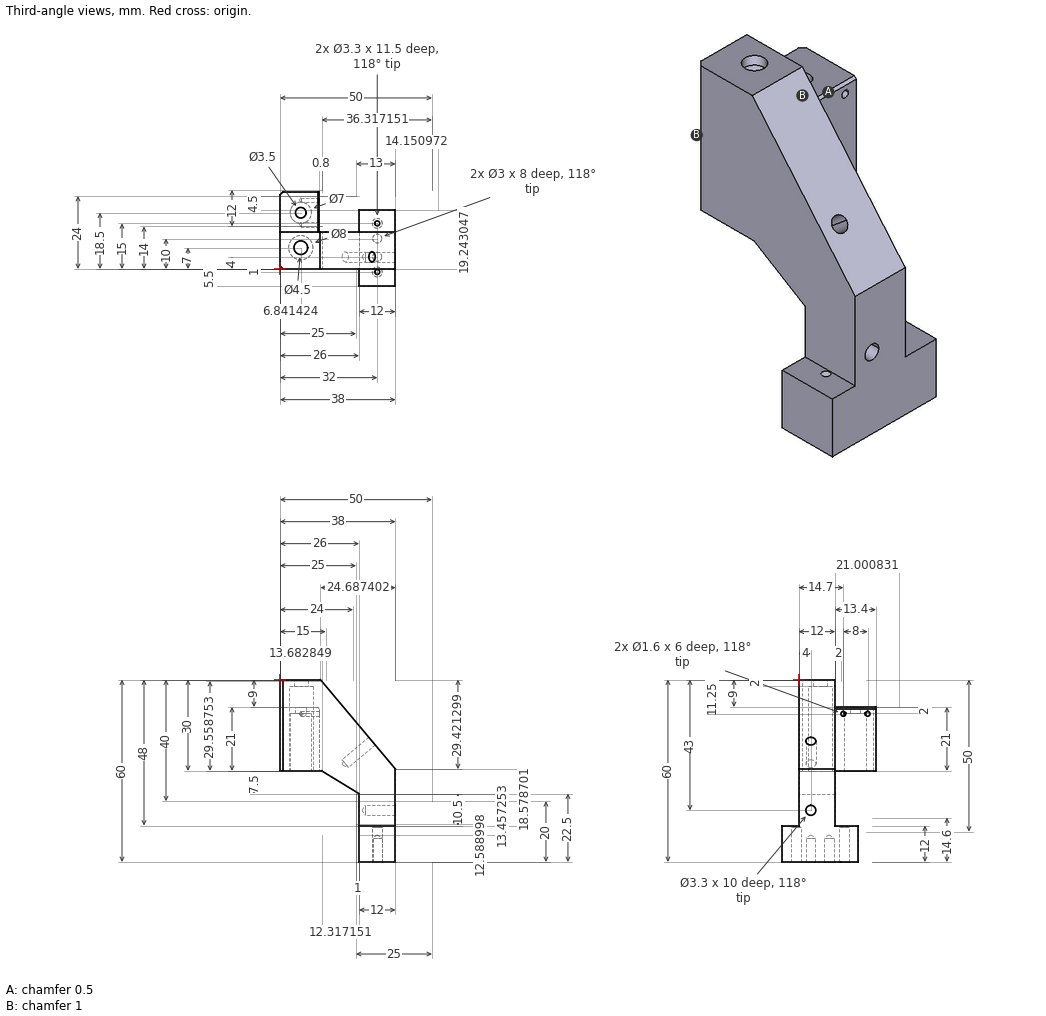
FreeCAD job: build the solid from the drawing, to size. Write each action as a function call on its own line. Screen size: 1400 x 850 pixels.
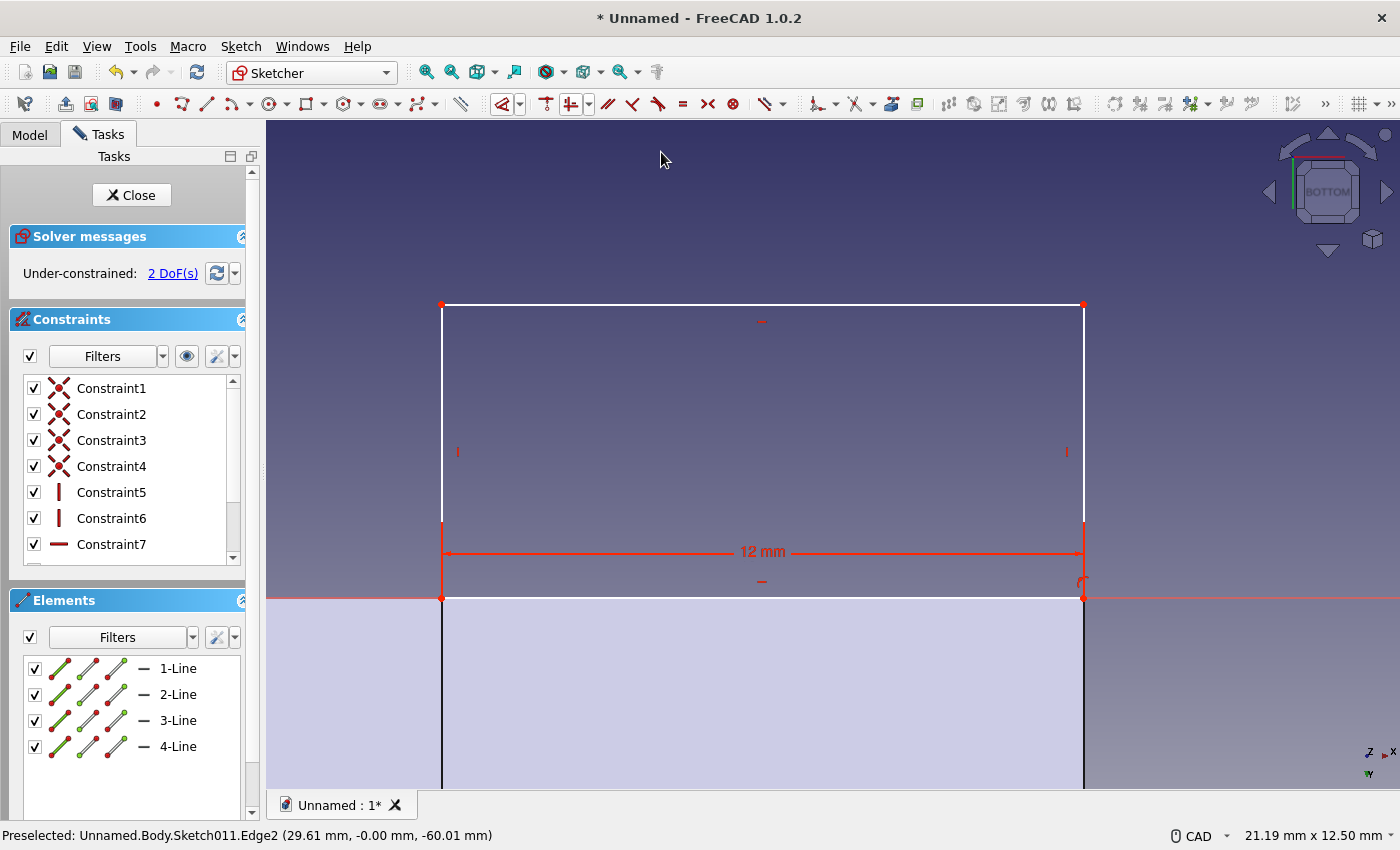
click(442, 393)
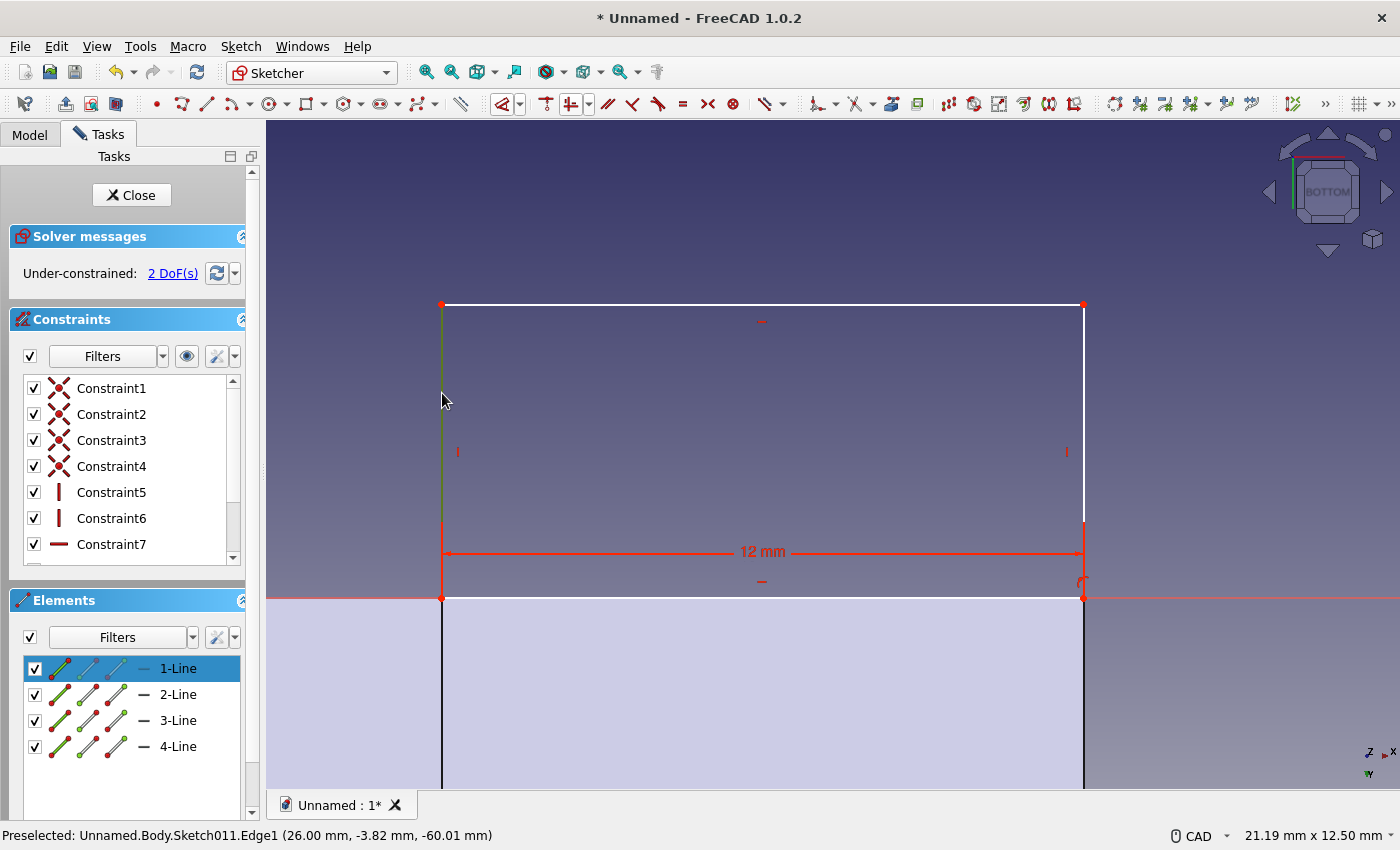
key(i)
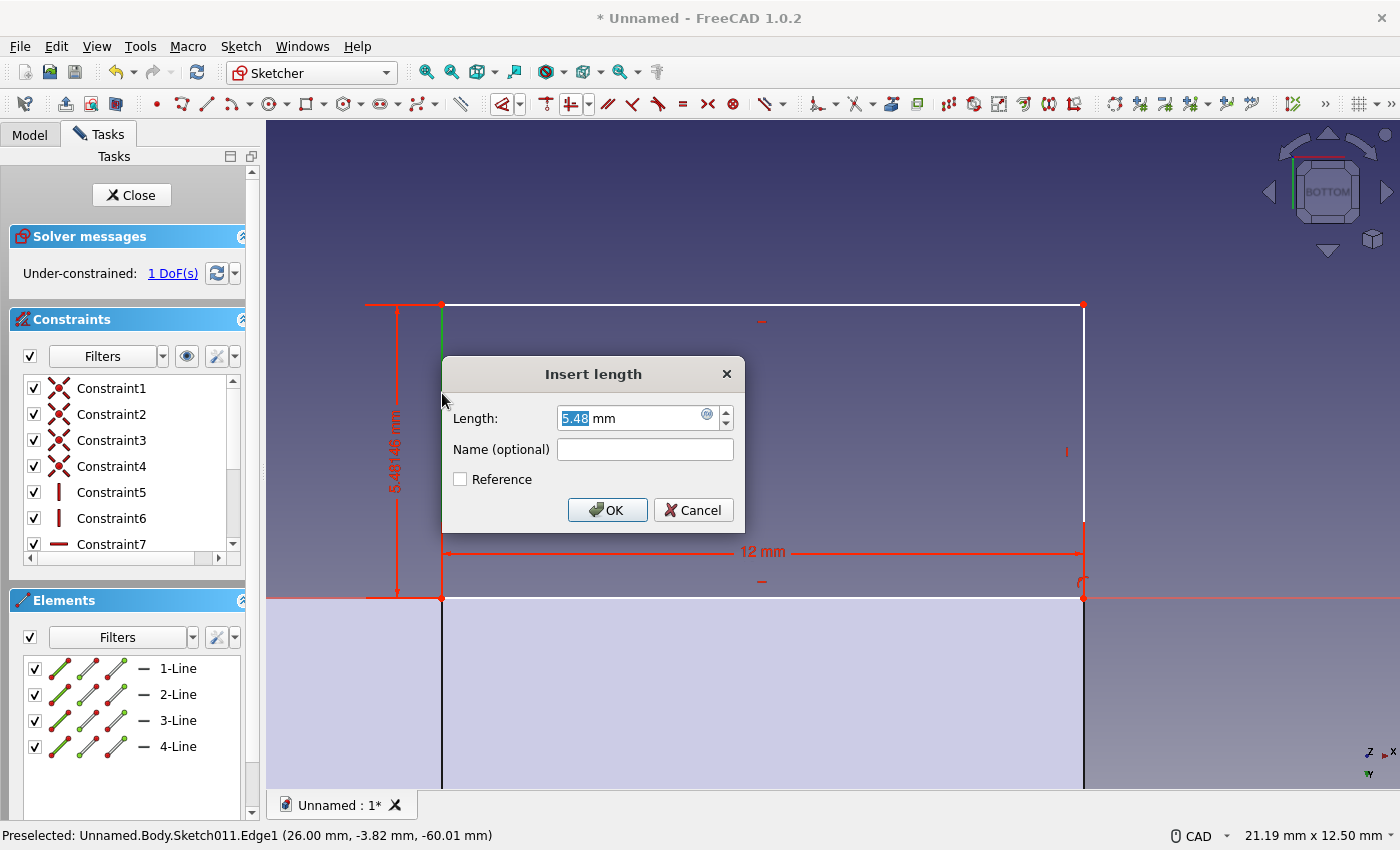
text(5.5)
key(Return)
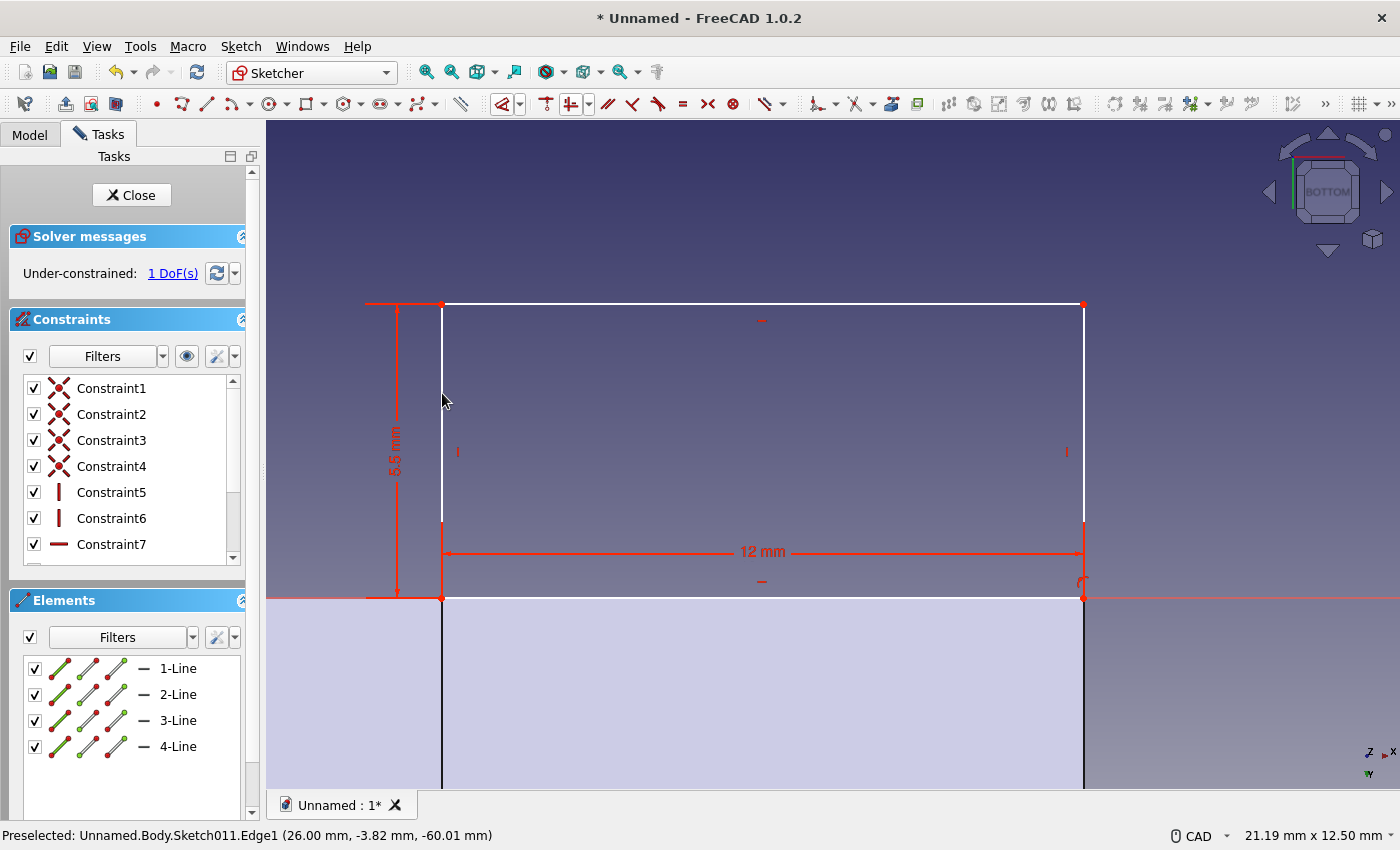
click(442, 304)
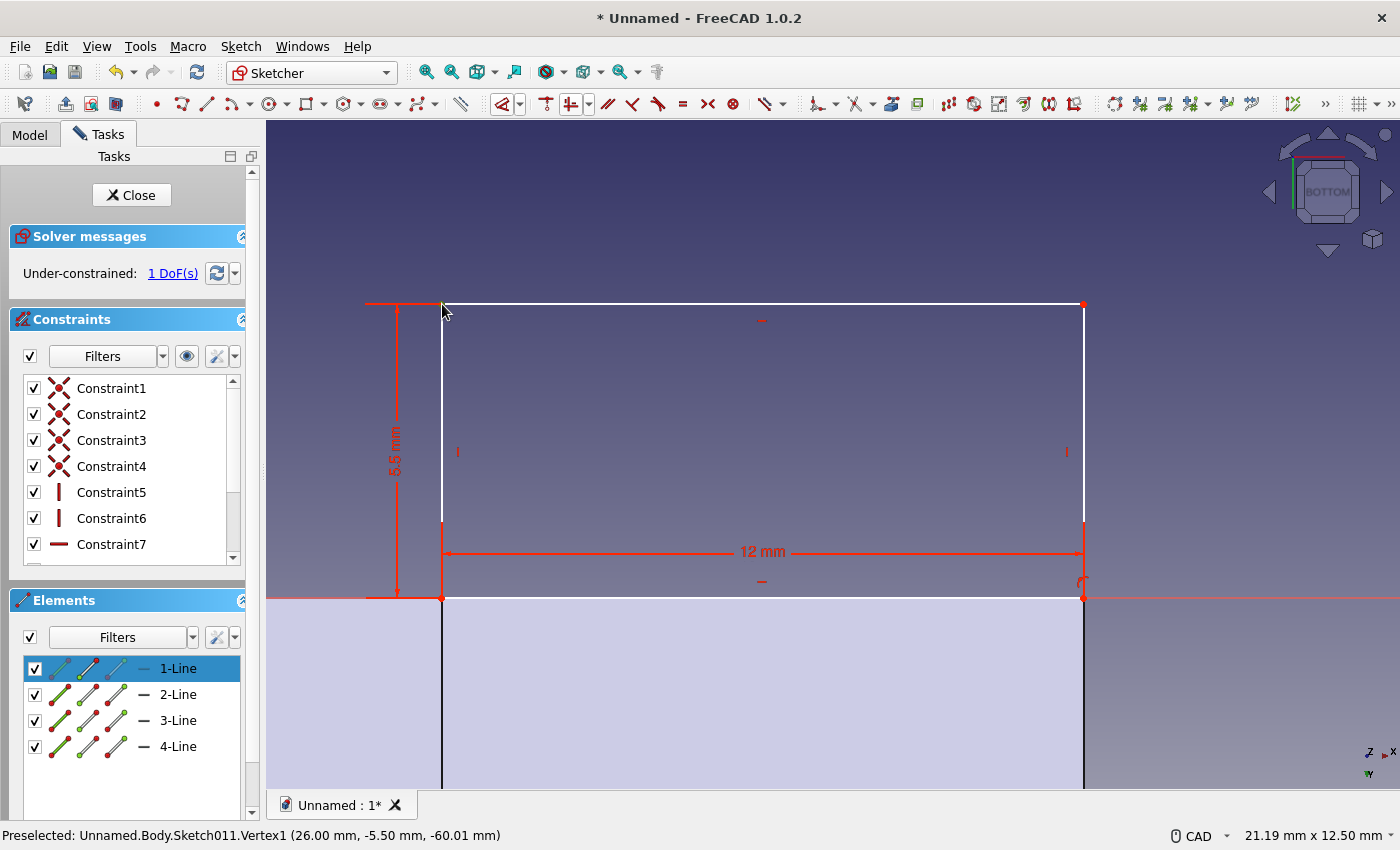
key(l)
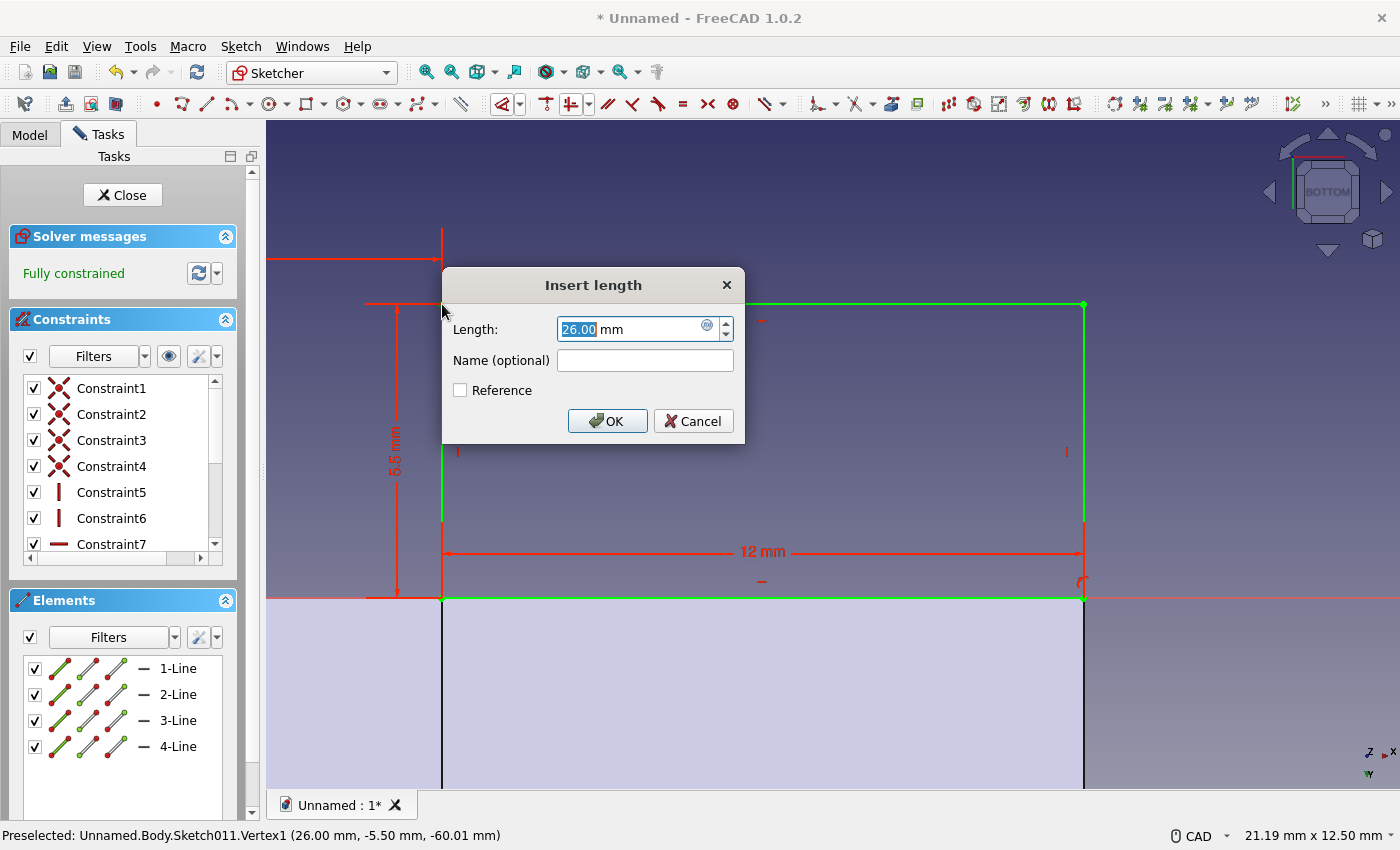
text(26)
key(Return)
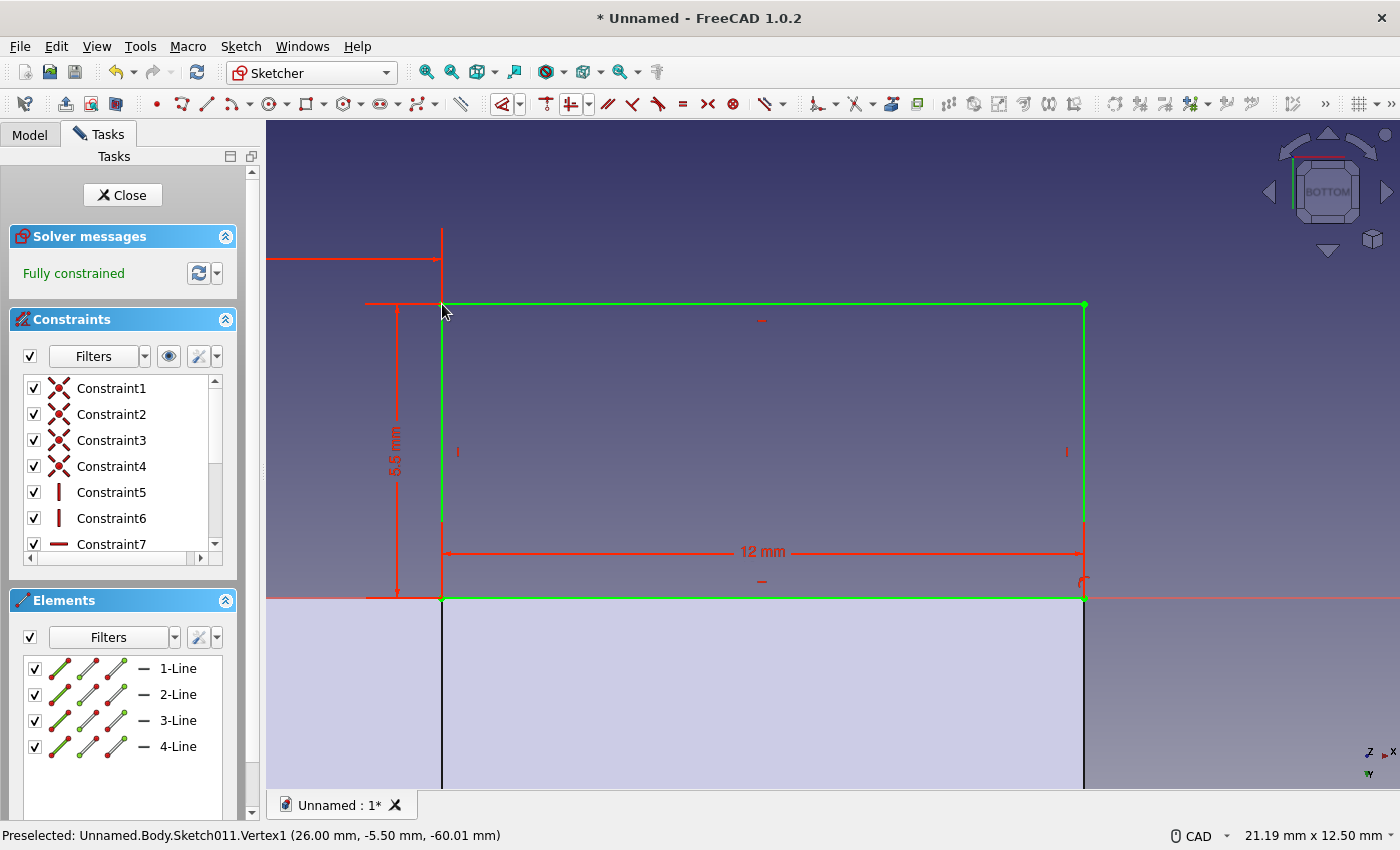
click(123, 195)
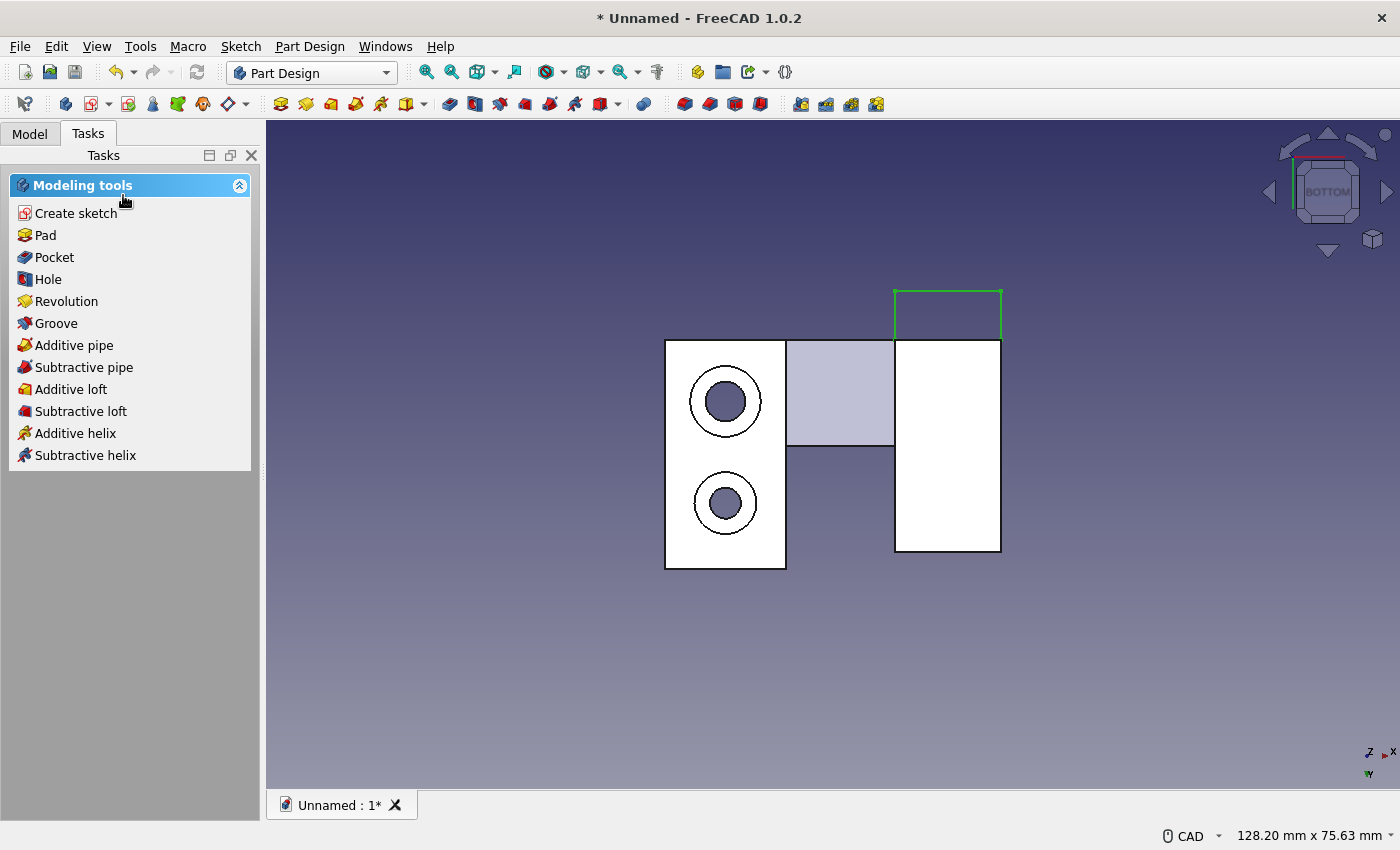
click(281, 104)